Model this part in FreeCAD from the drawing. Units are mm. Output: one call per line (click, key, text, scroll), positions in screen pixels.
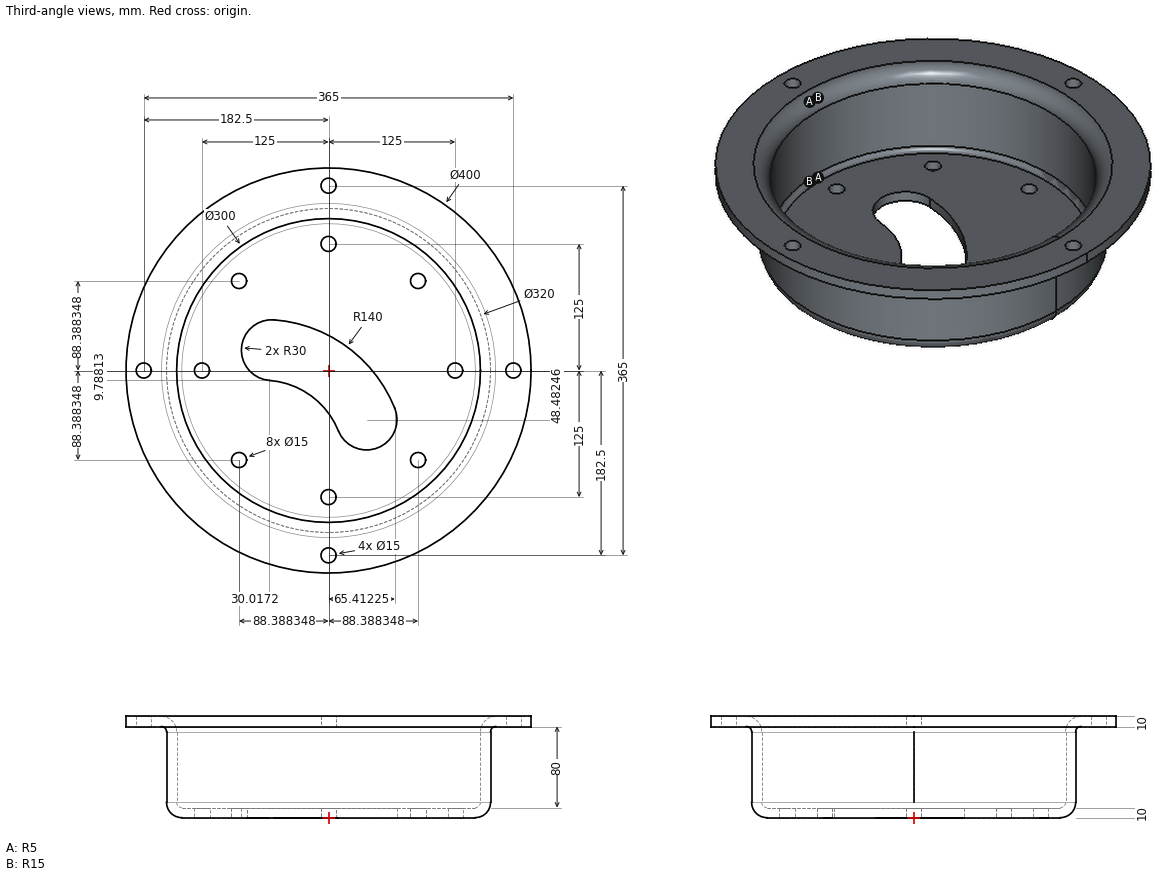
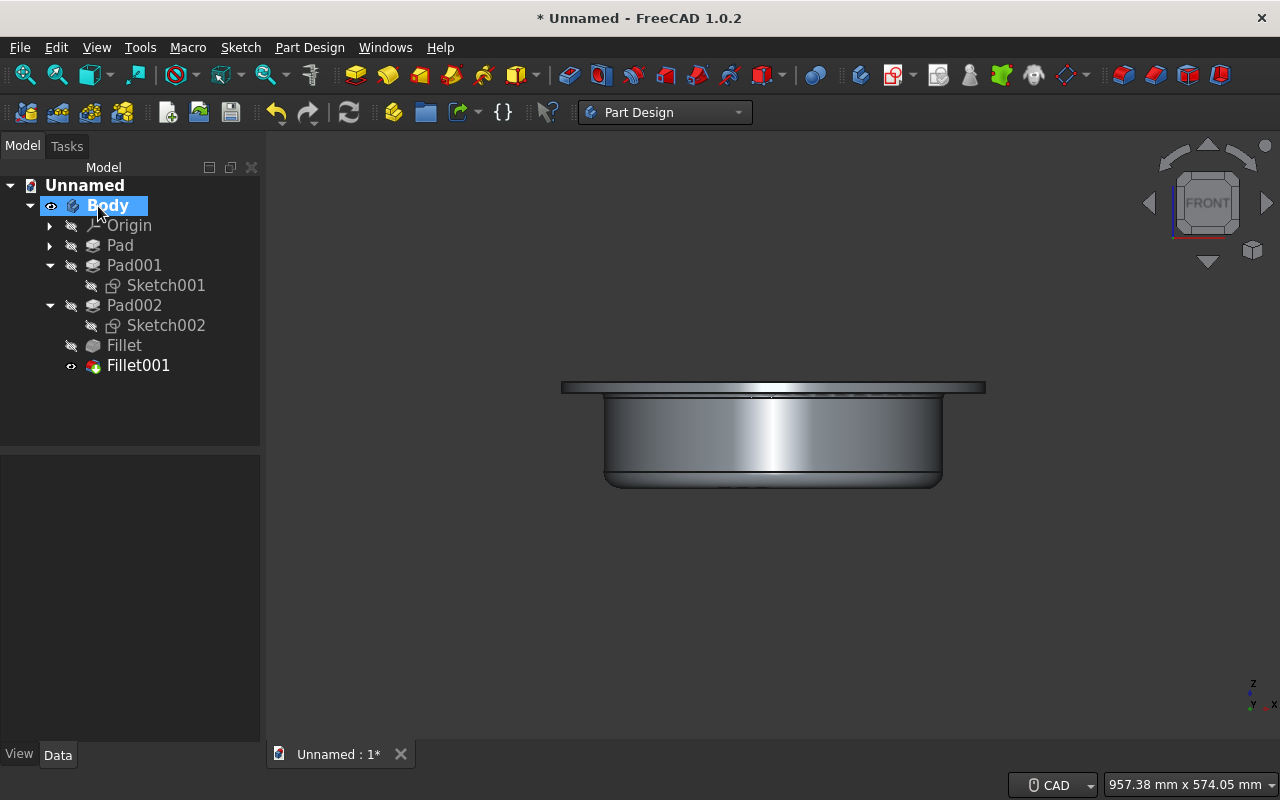
key(0)